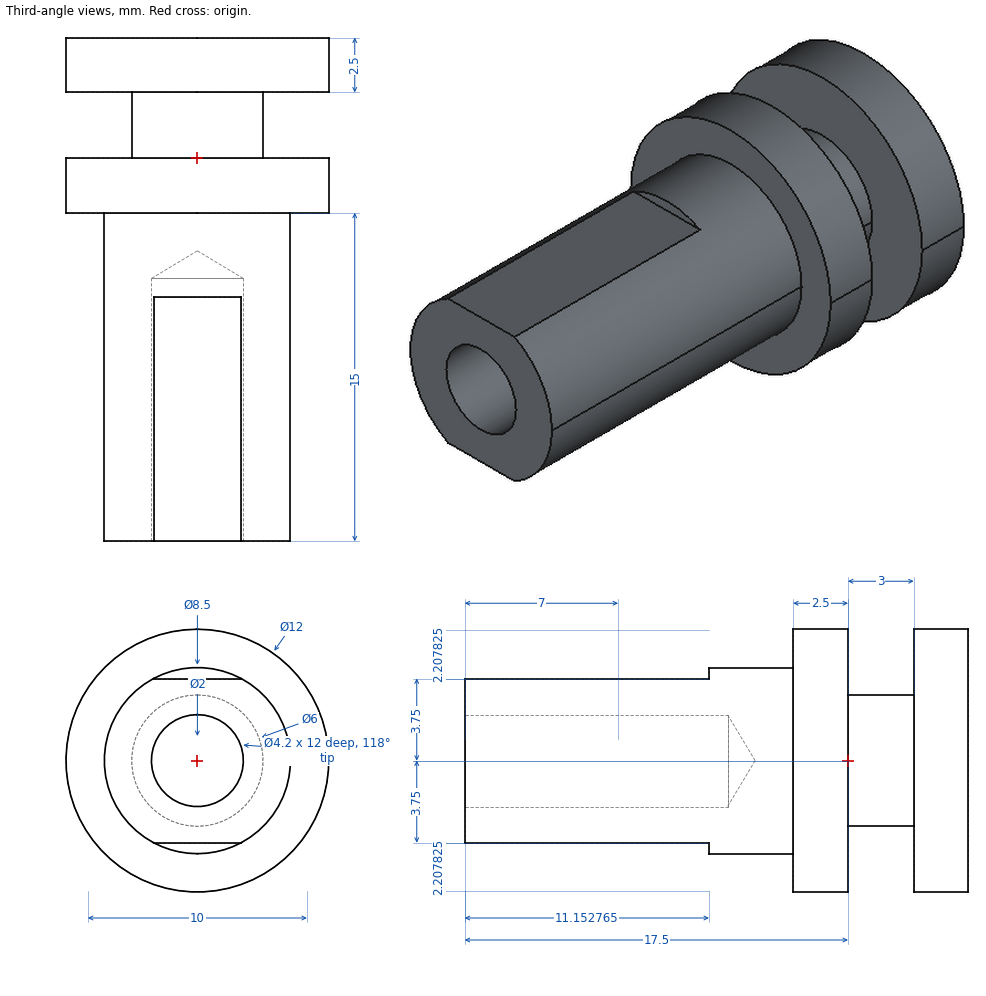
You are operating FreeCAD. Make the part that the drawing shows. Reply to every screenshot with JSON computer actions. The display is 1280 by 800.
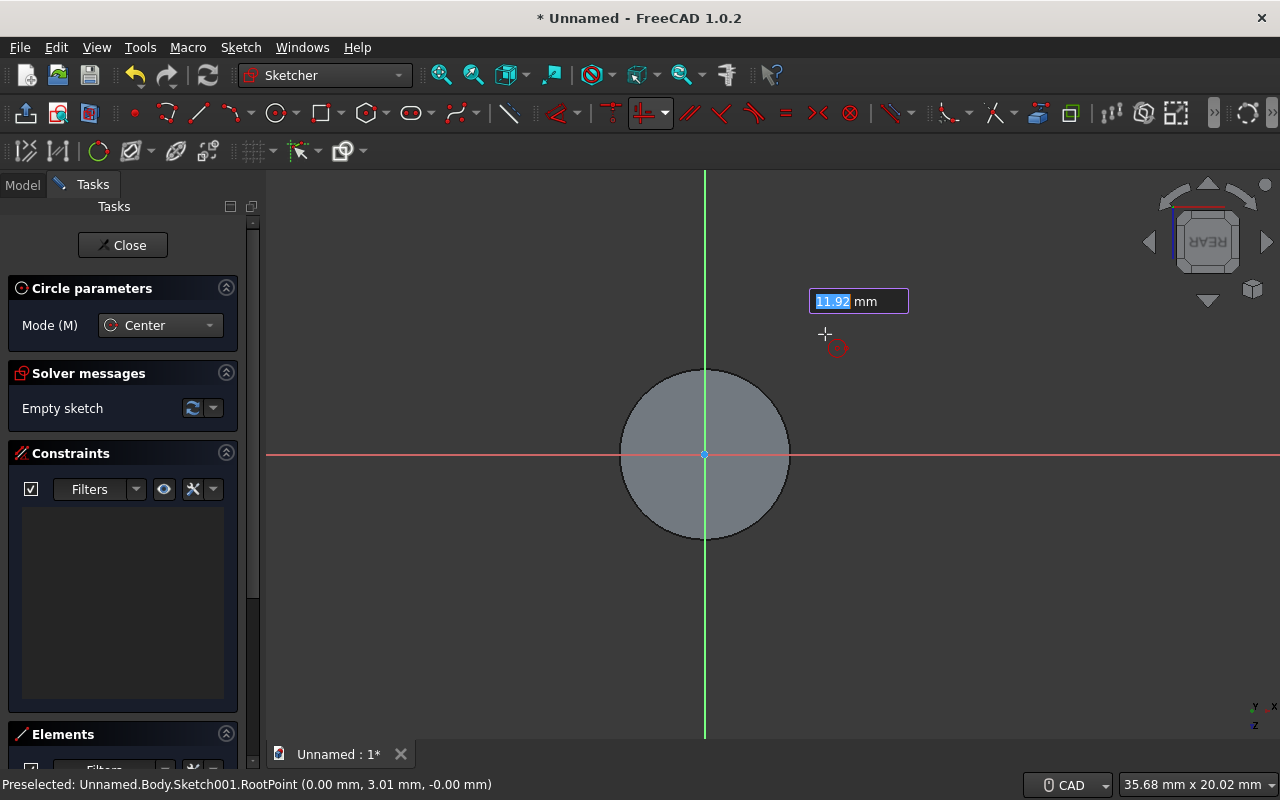
{"action": "type", "text": "12"}
{"action": "key", "text": "Return"}
{"action": "key", "text": "Escape"}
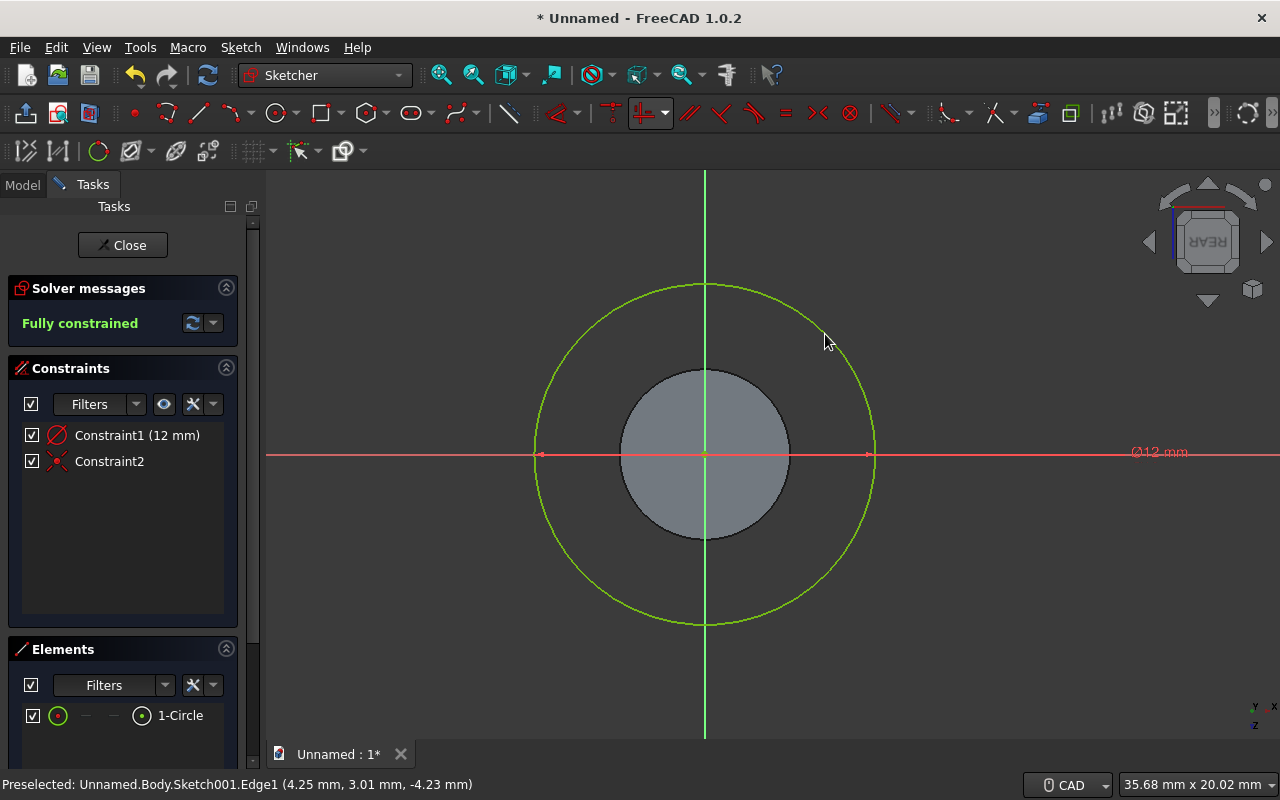
{"action": "left_click", "coordinate": [123, 245]}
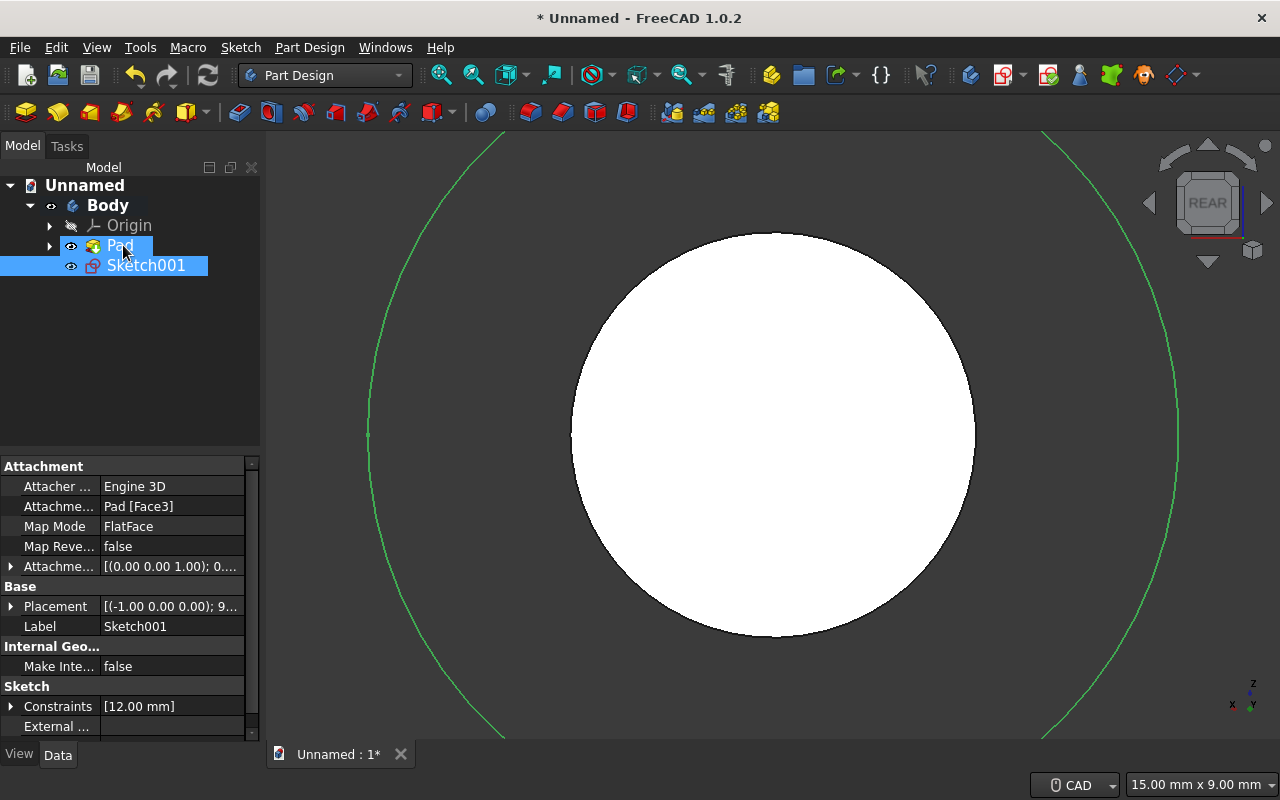
{"action": "left_click", "coordinate": [26, 112]}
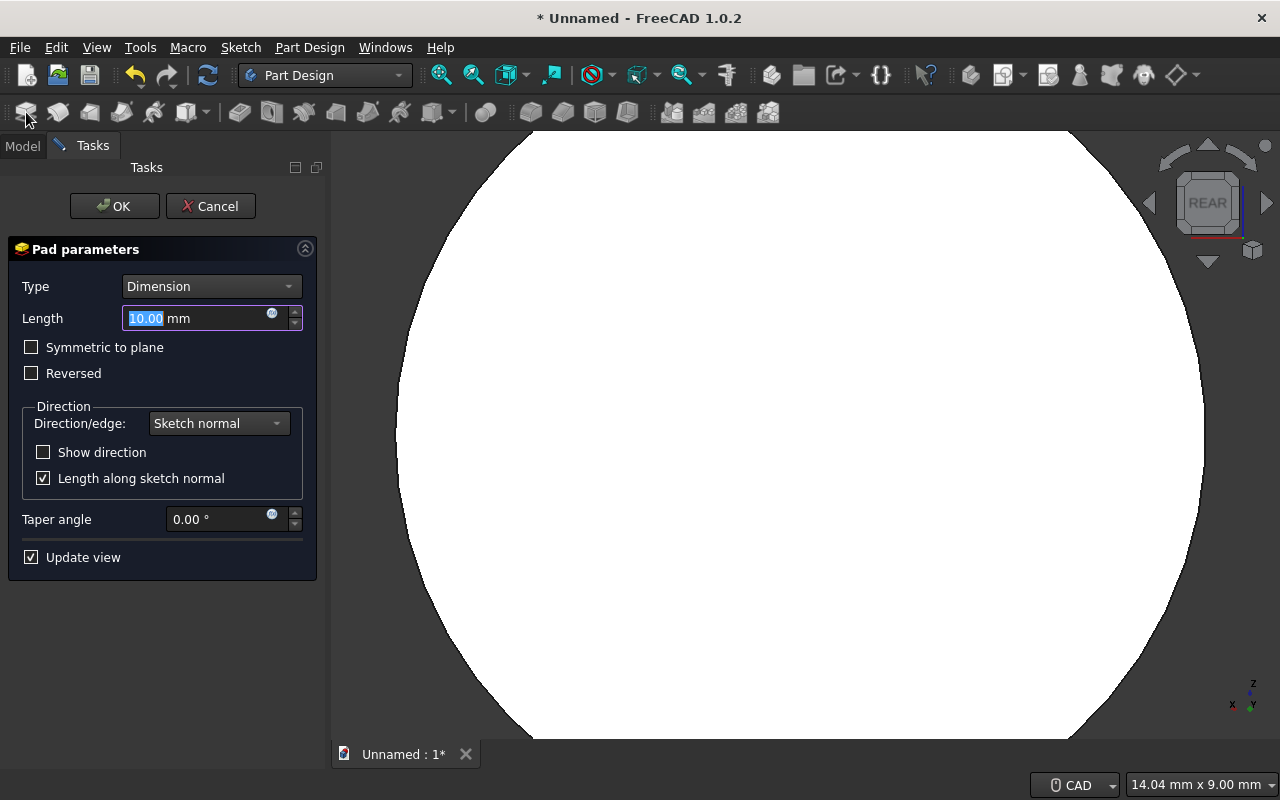
{"action": "type", "text": "2.5"}
{"action": "key", "text": "Tab"}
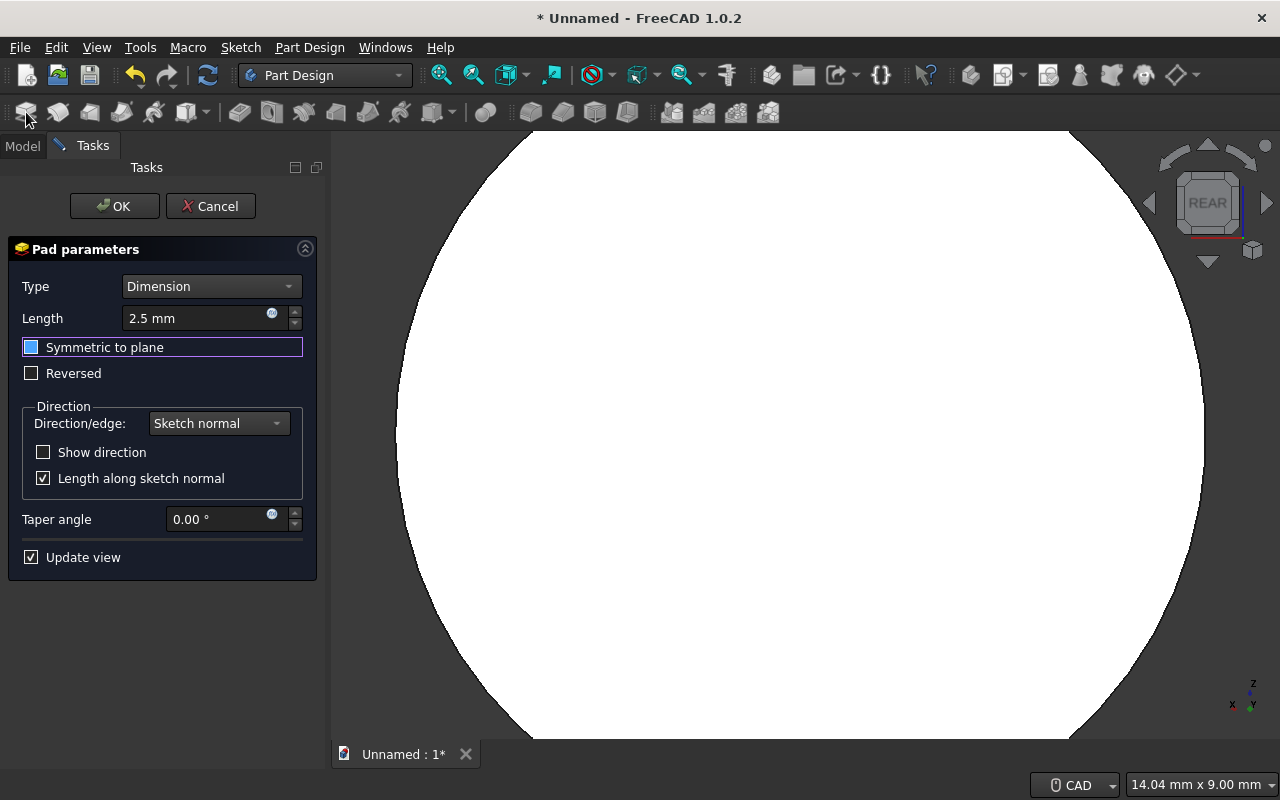
{"action": "left_click", "coordinate": [115, 206]}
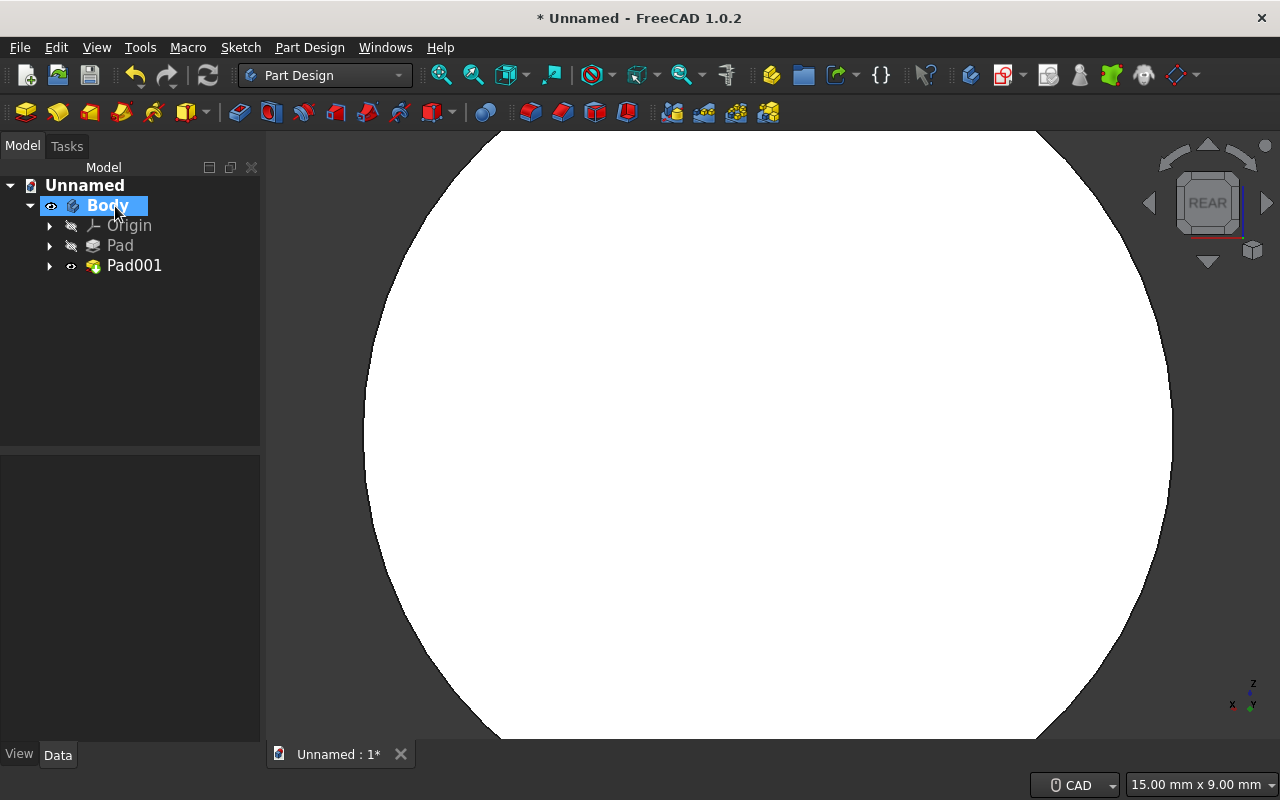
{"action": "key", "text": "v f"}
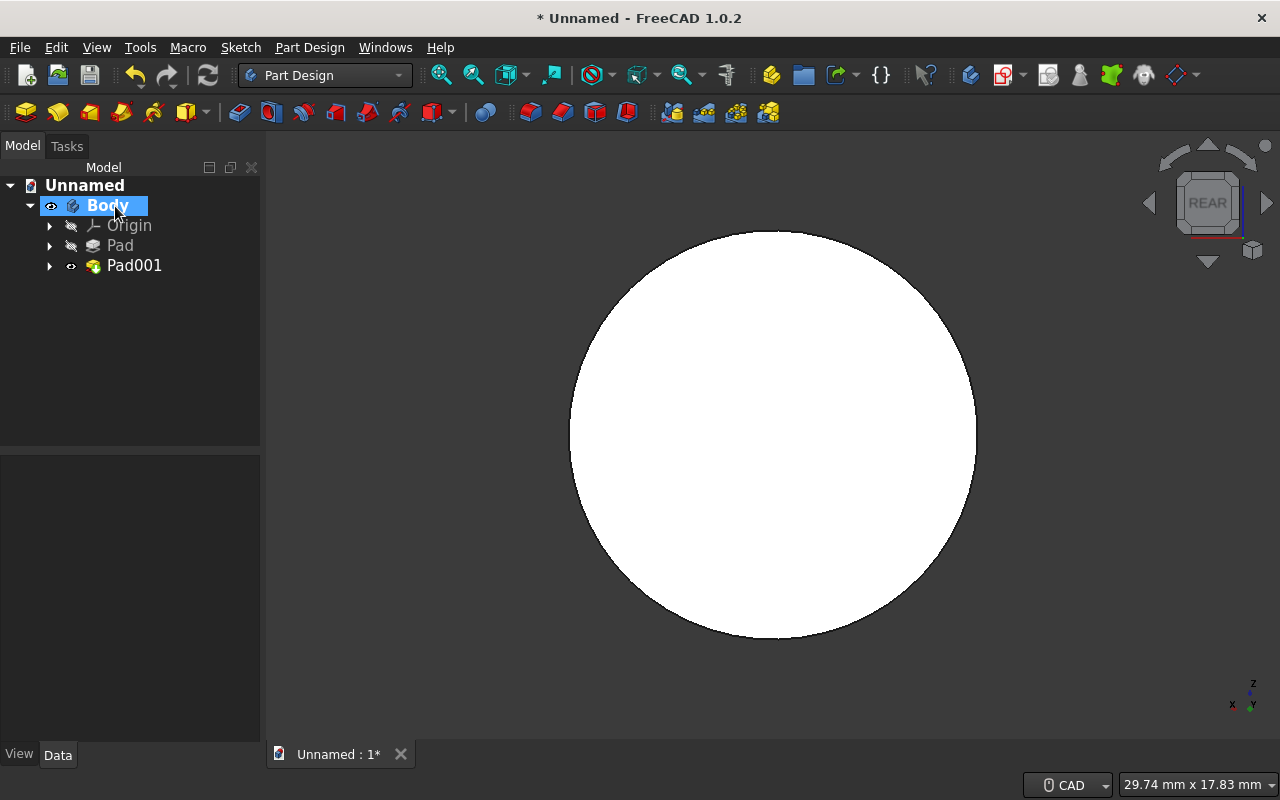
{"action": "left_click", "coordinate": [50, 226]}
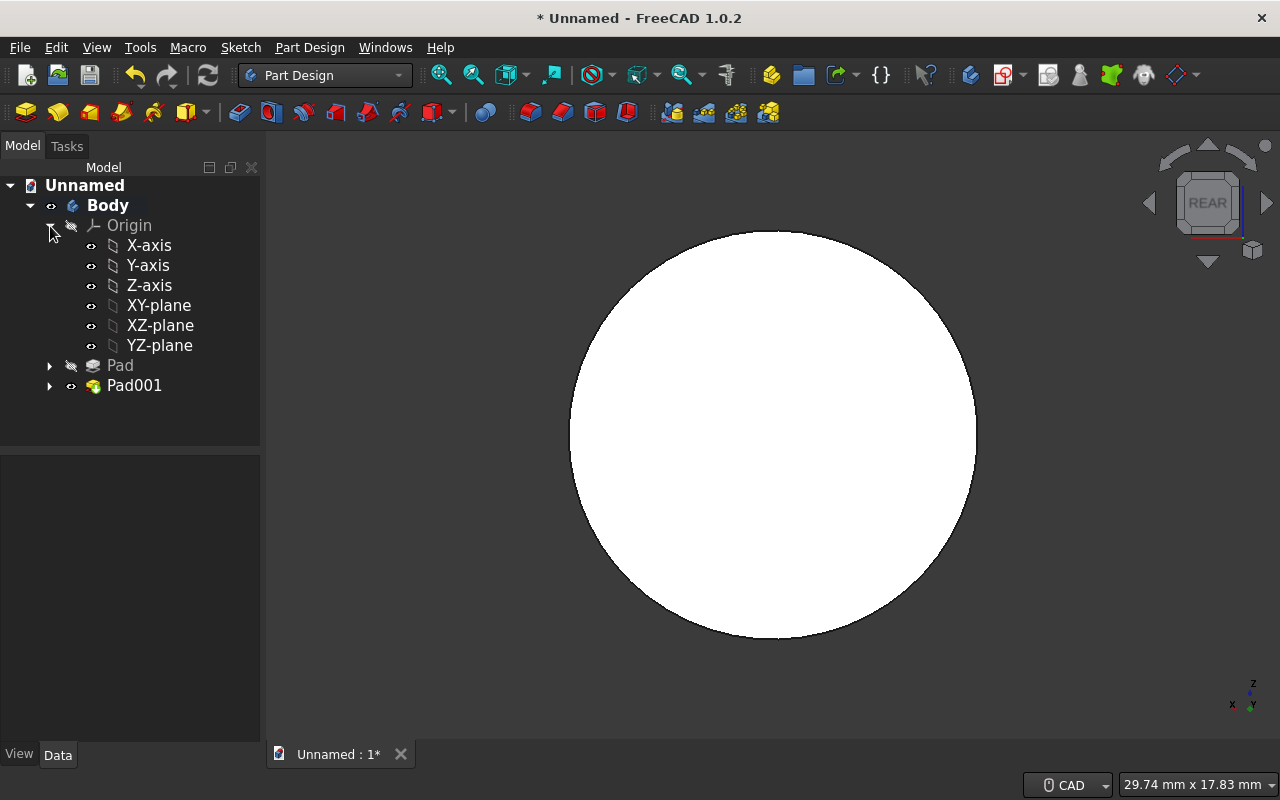
{"action": "left_click", "coordinate": [136, 326]}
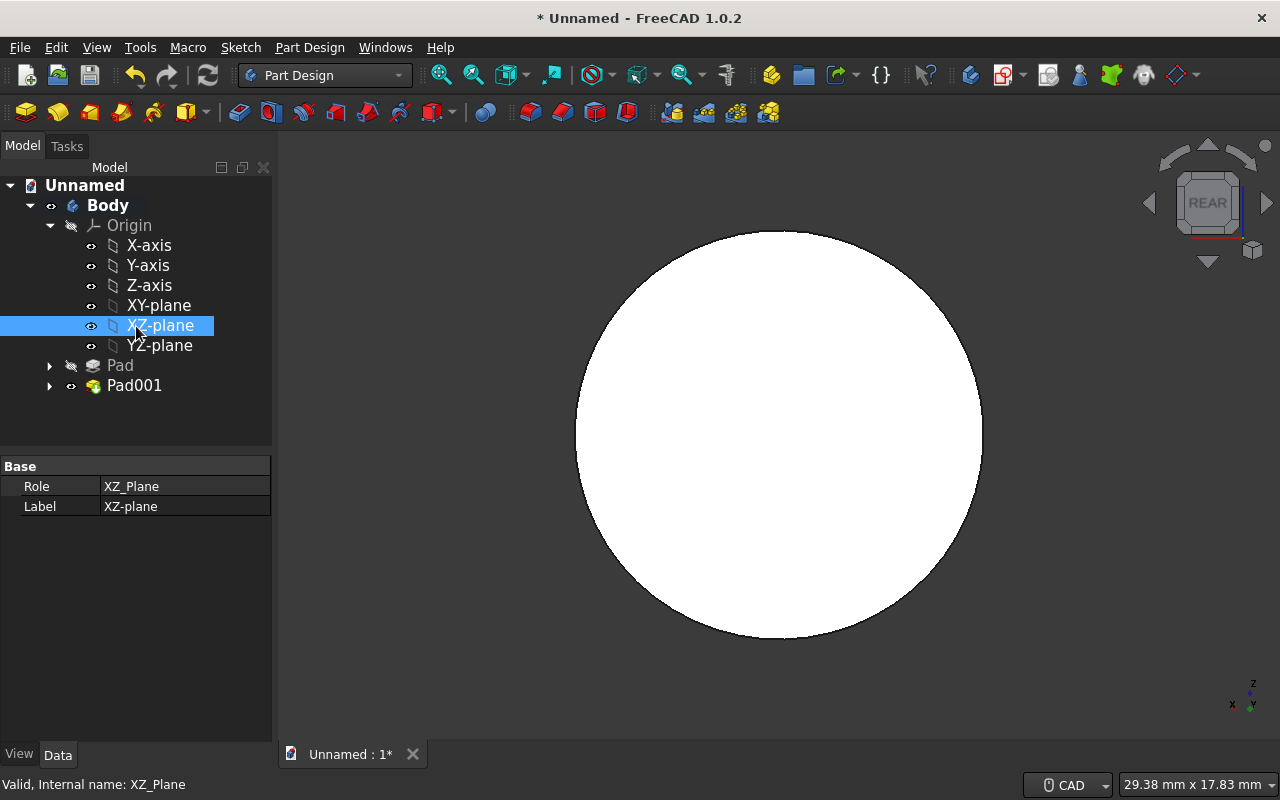
{"action": "left_click", "coordinate": [1176, 76]}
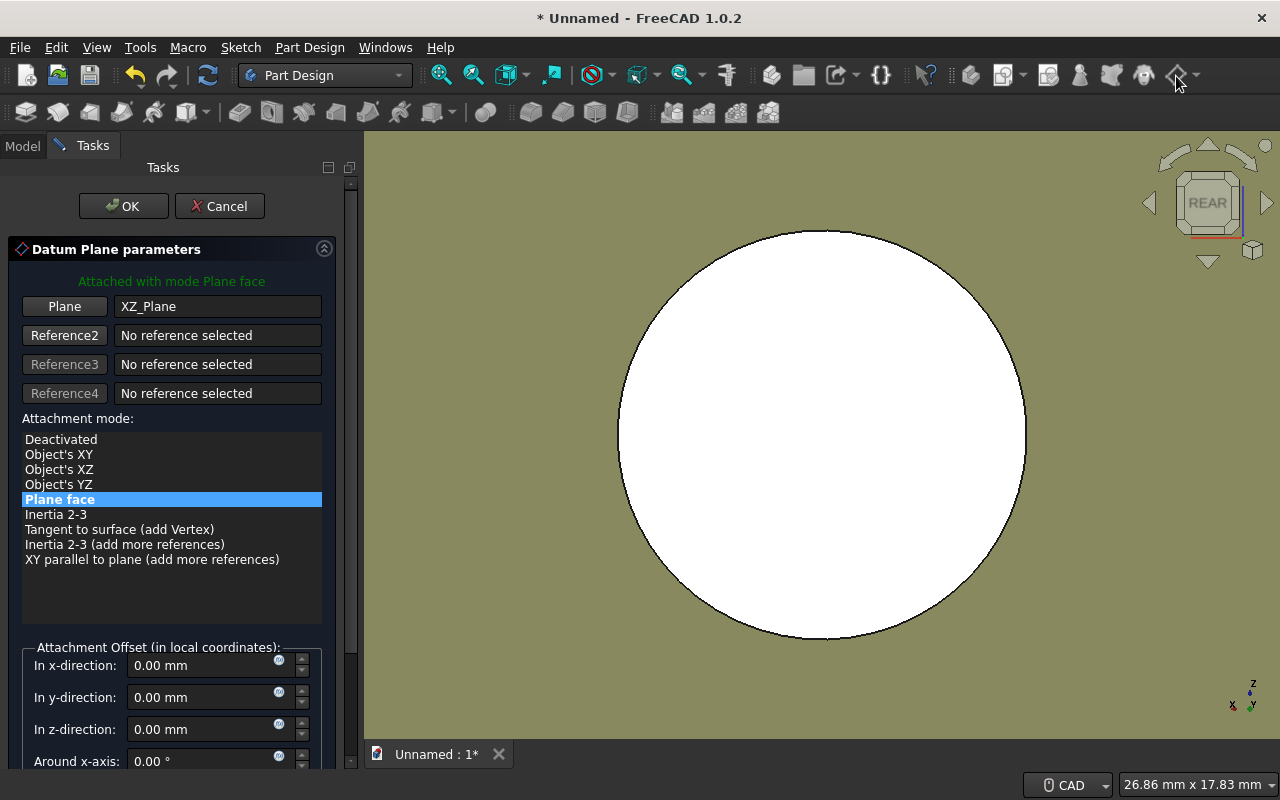
{"action": "triple_click", "coordinate": [210, 729]}